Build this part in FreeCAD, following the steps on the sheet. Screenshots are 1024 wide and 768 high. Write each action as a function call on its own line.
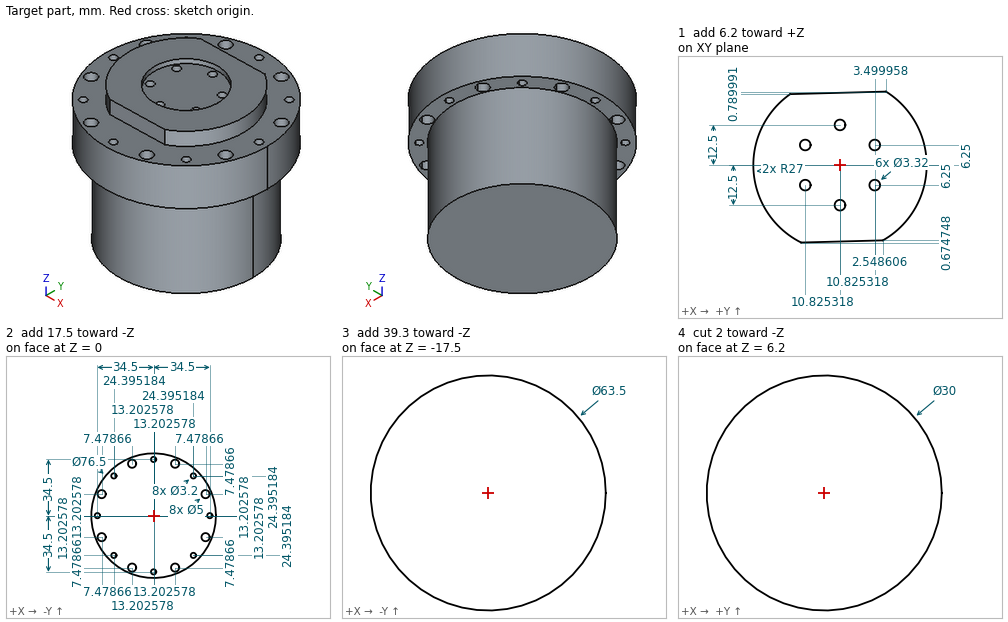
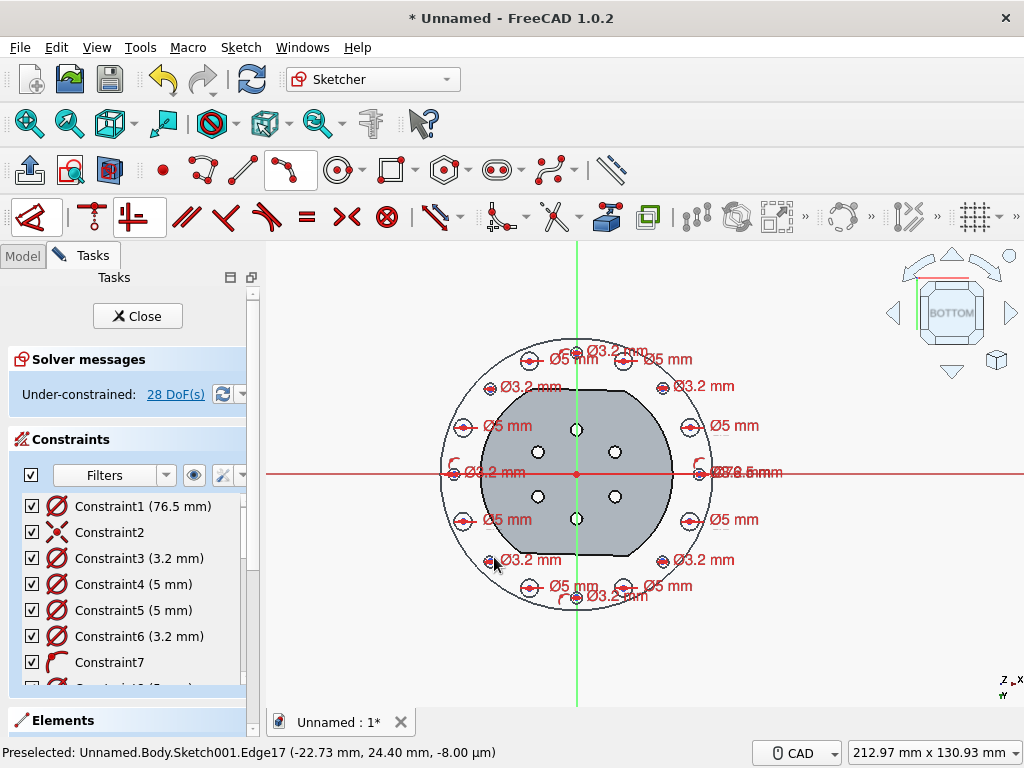
click(624, 361)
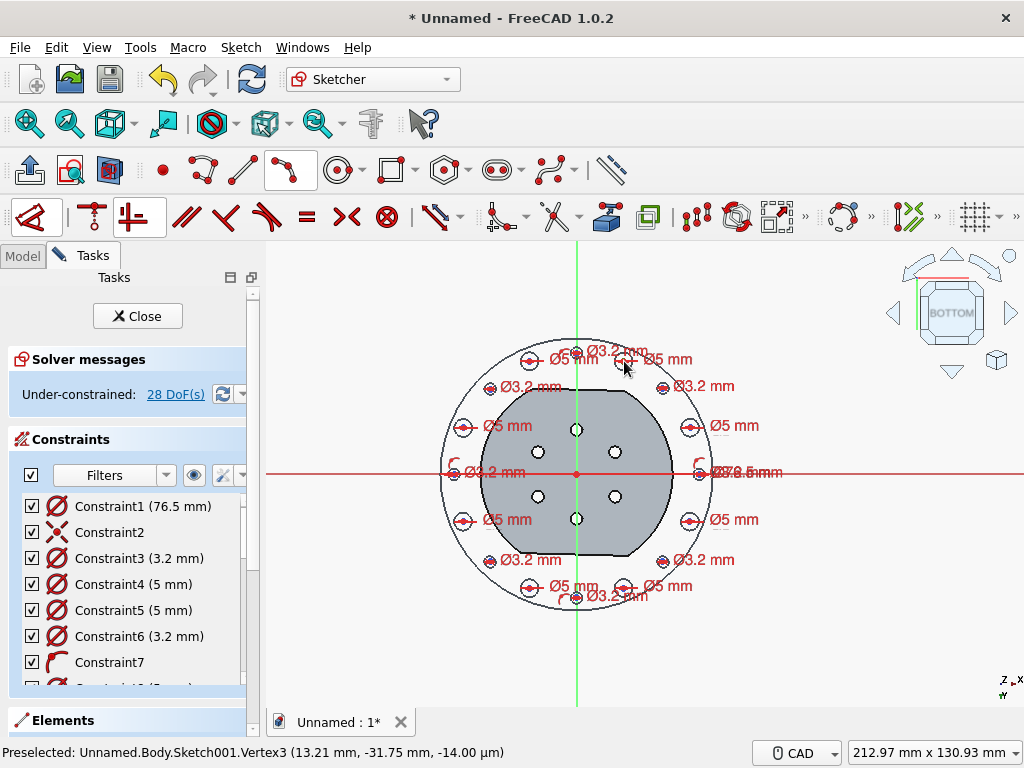
click(530, 361)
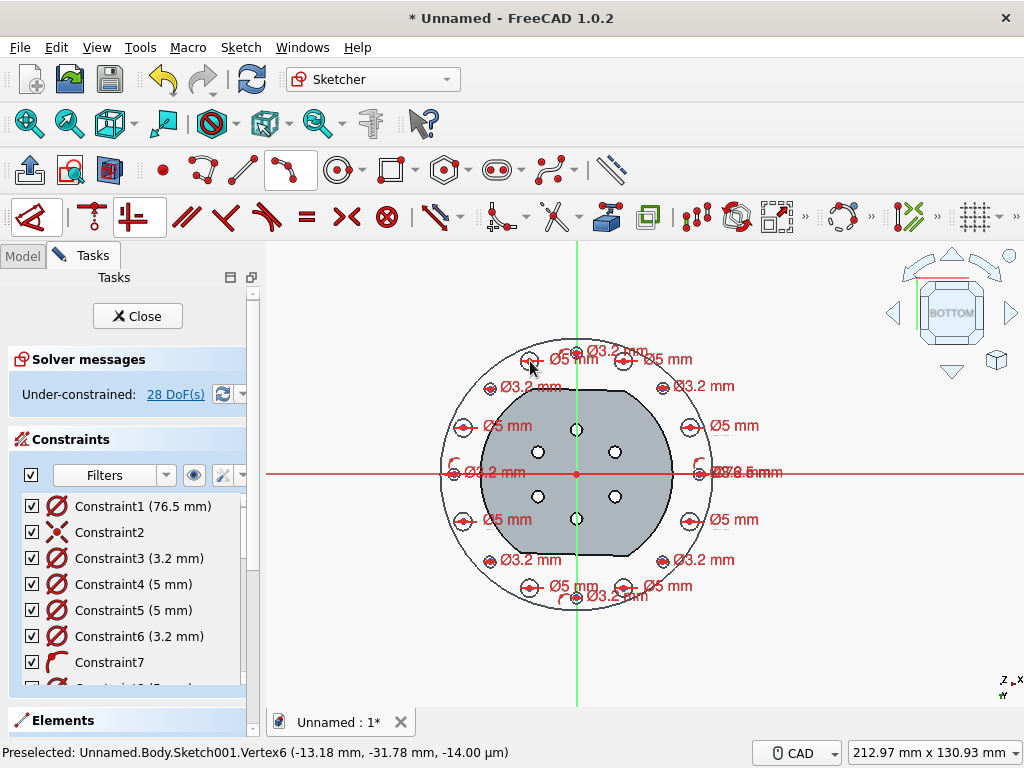
click(160, 218)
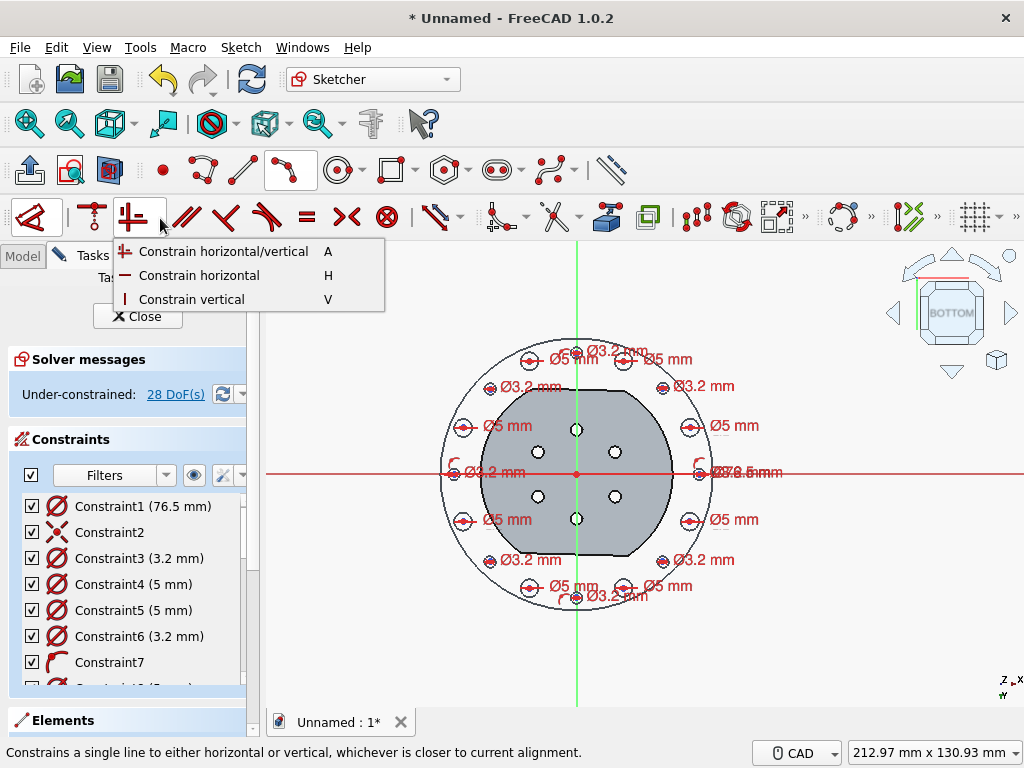
click(249, 275)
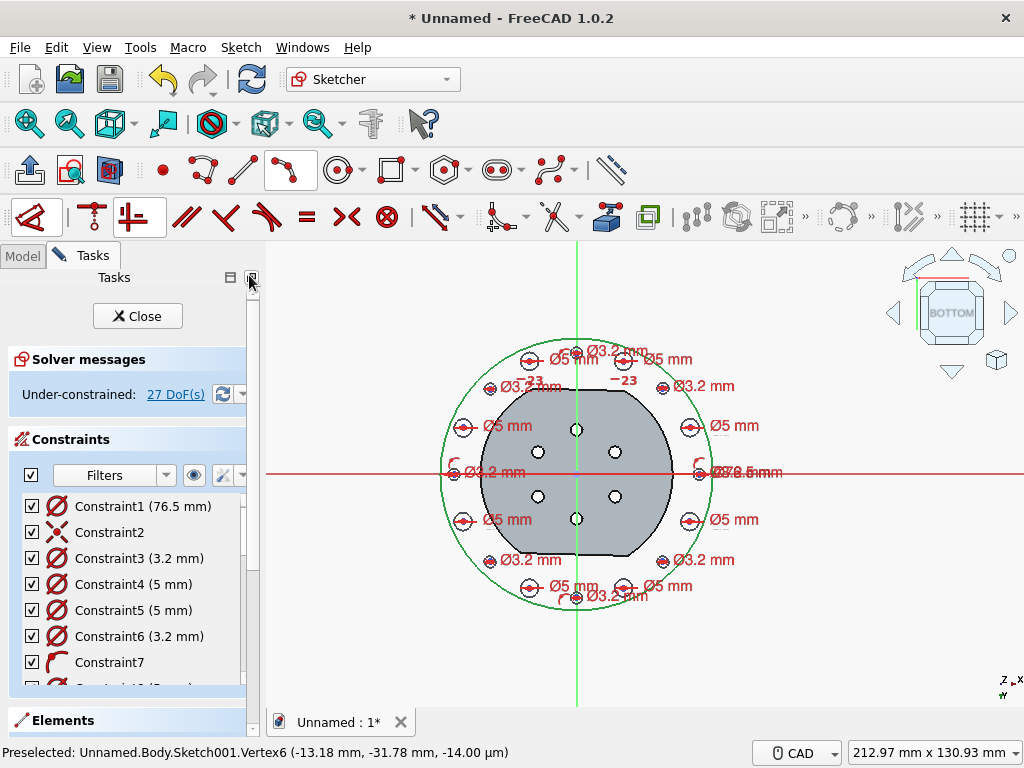
click(663, 388)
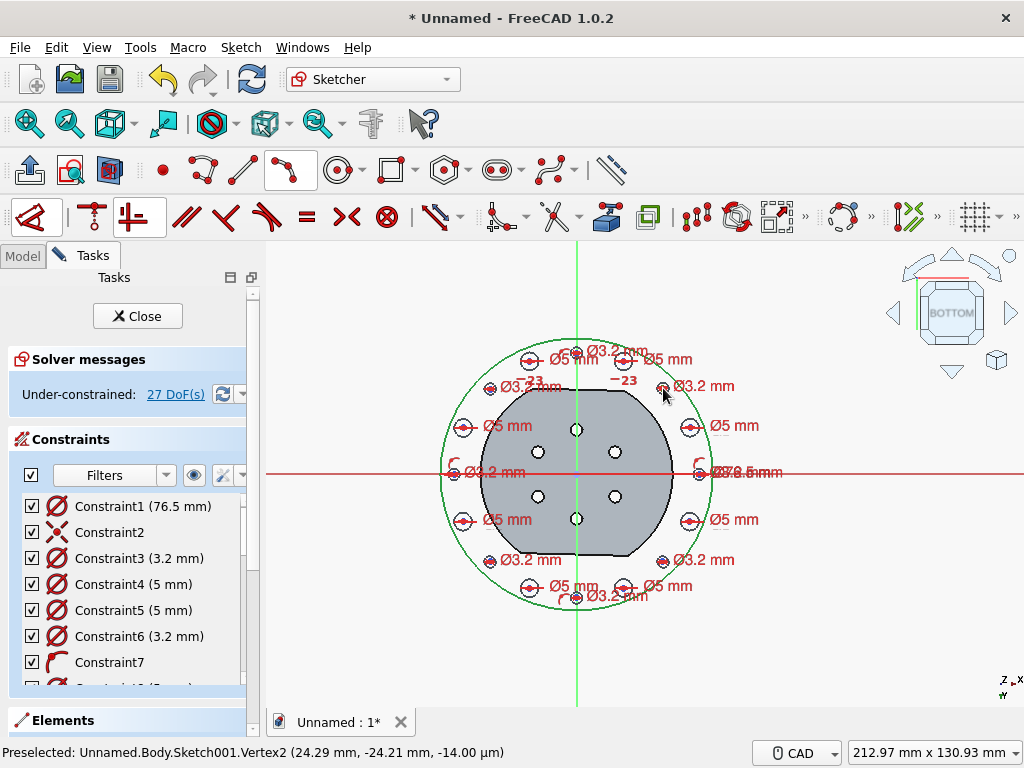
click(490, 389)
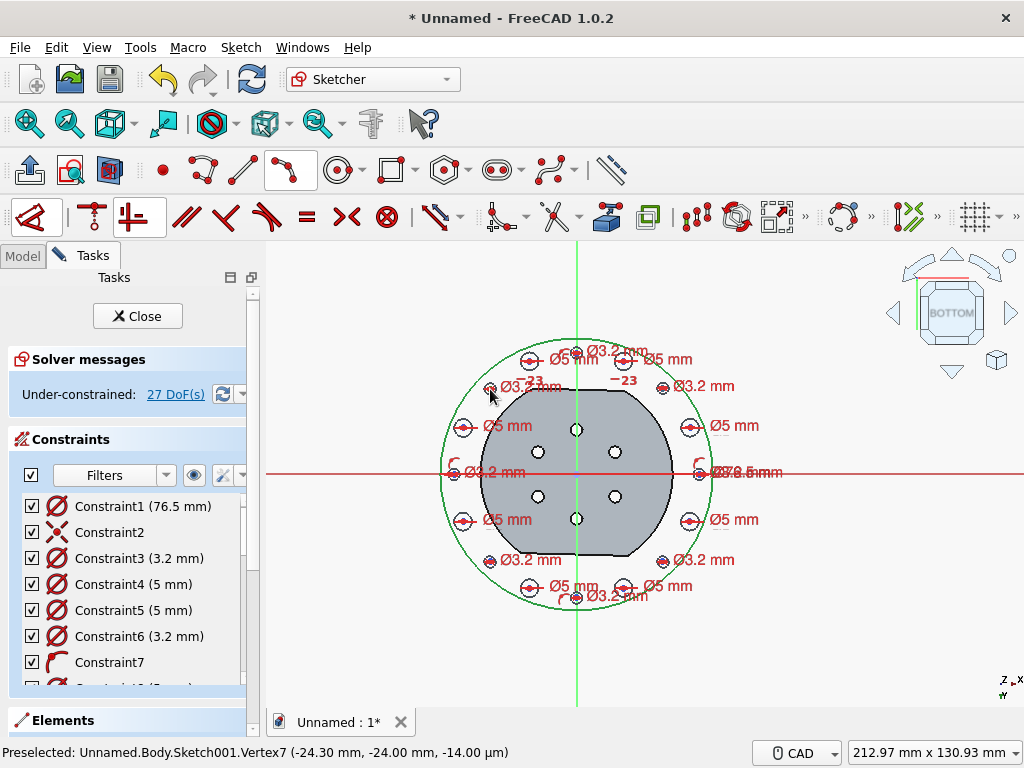
click(160, 218)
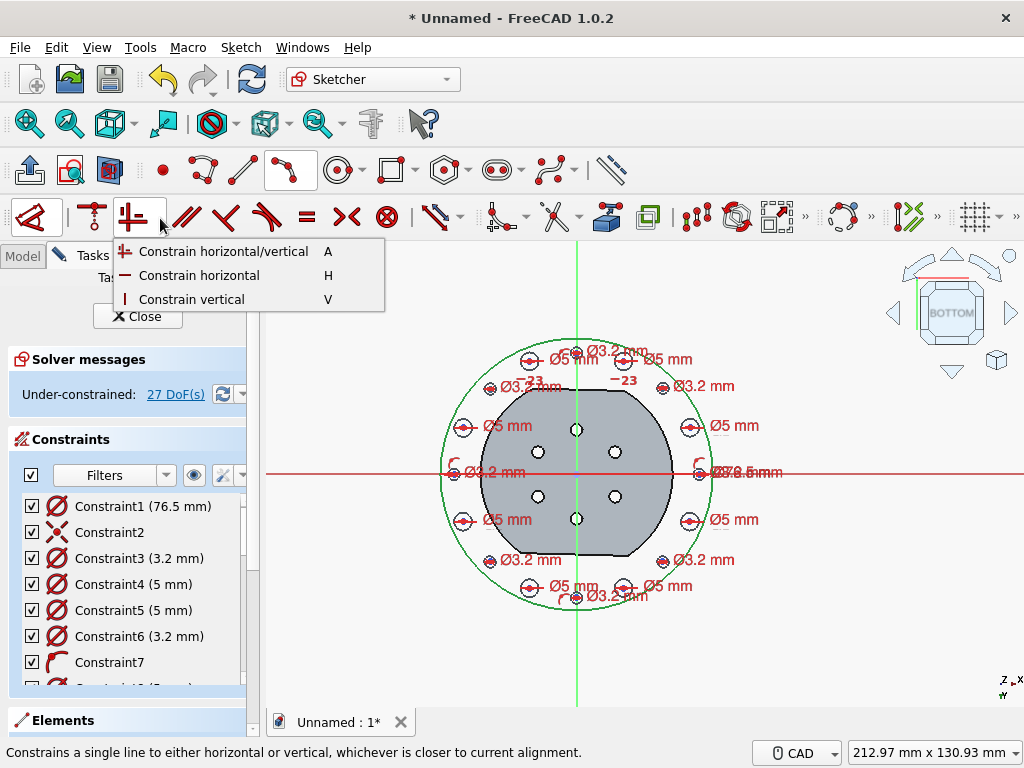
click(249, 275)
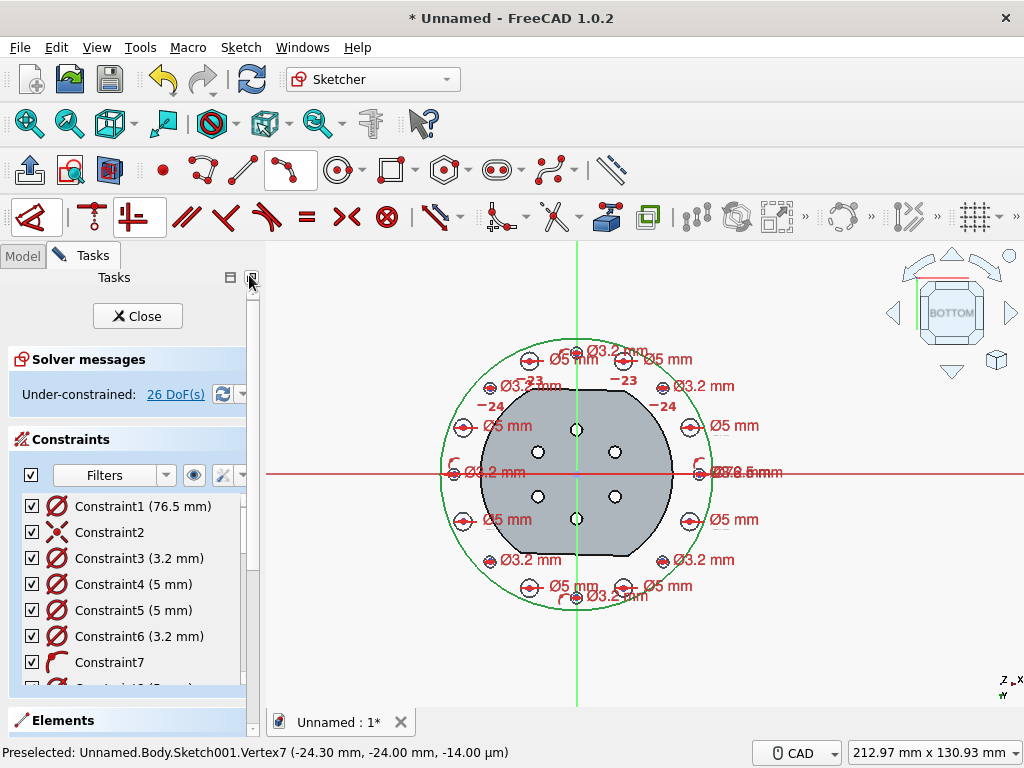
click(690, 428)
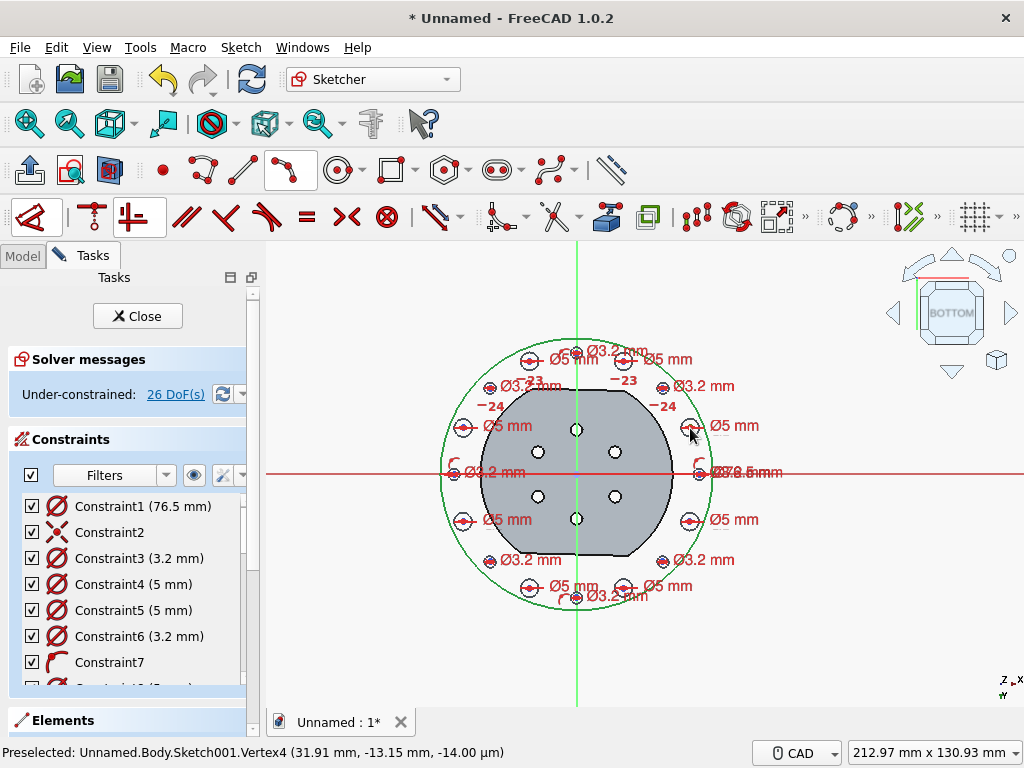
click(690, 522)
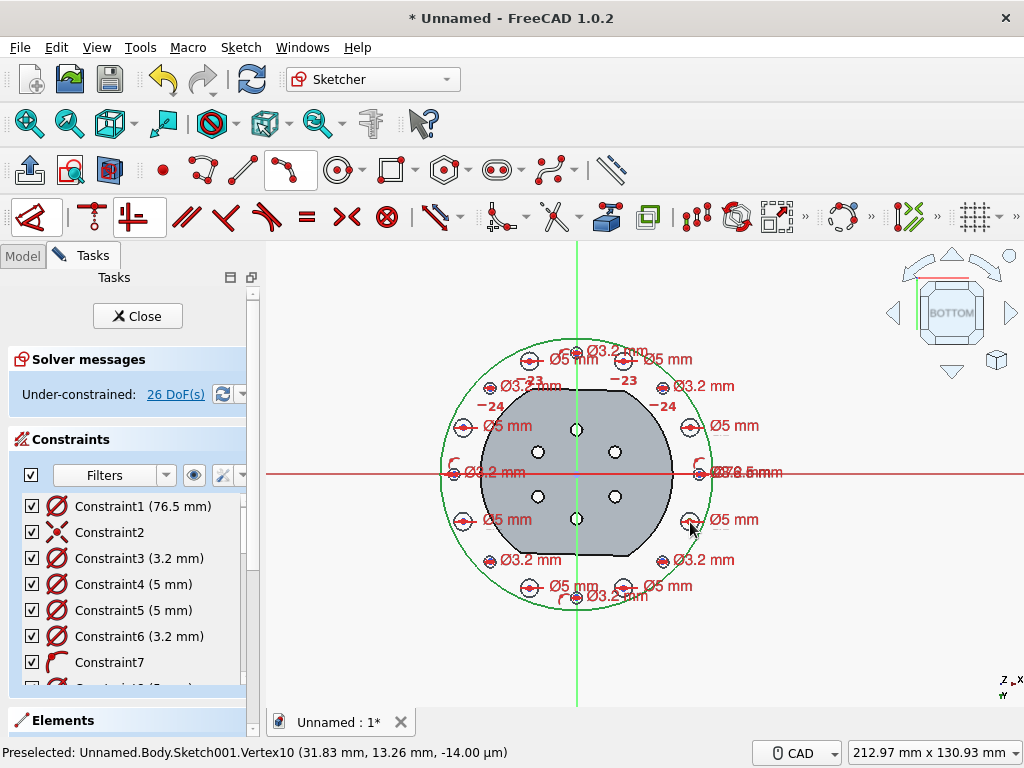
key(v)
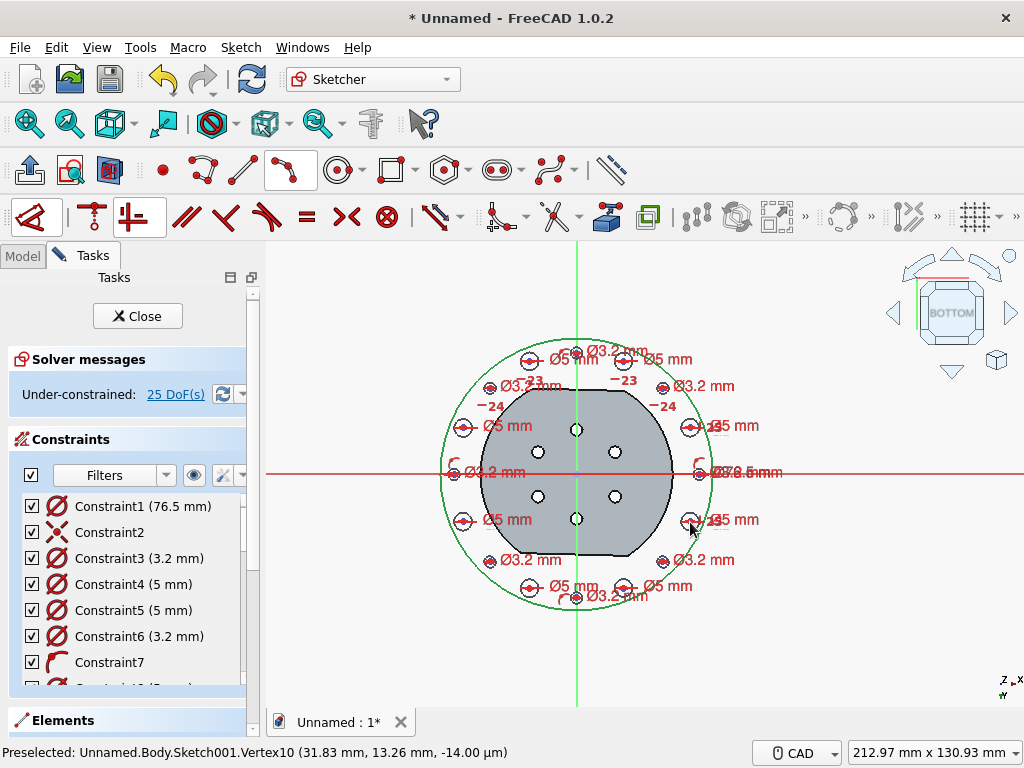
click(663, 388)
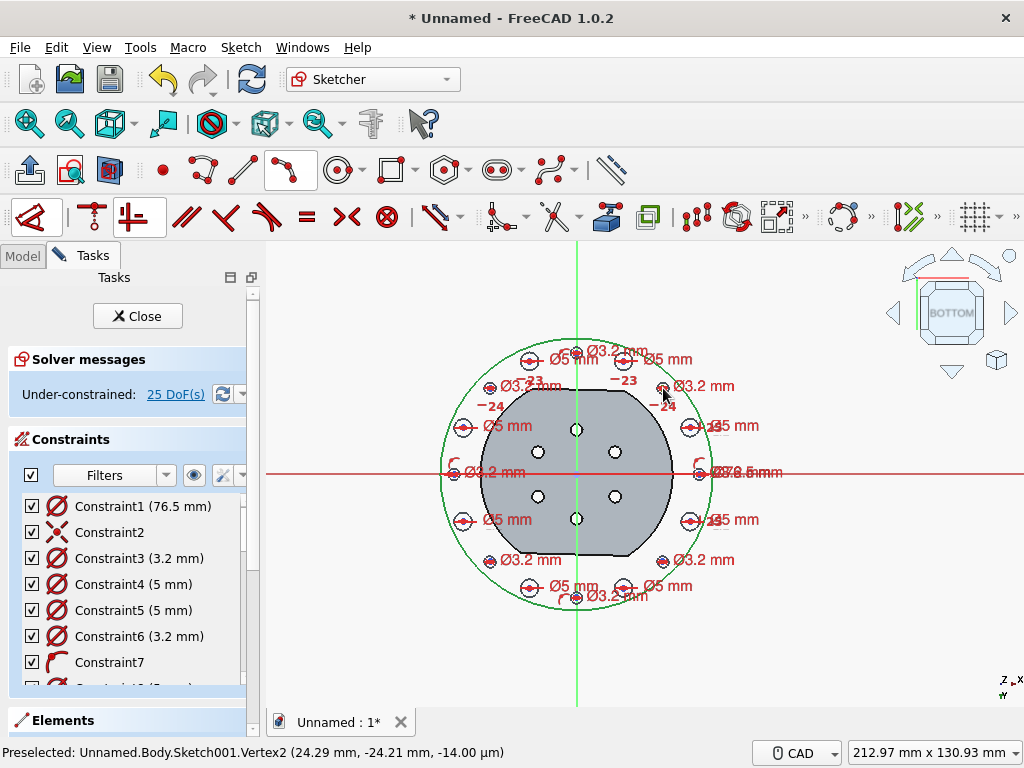
click(663, 562)